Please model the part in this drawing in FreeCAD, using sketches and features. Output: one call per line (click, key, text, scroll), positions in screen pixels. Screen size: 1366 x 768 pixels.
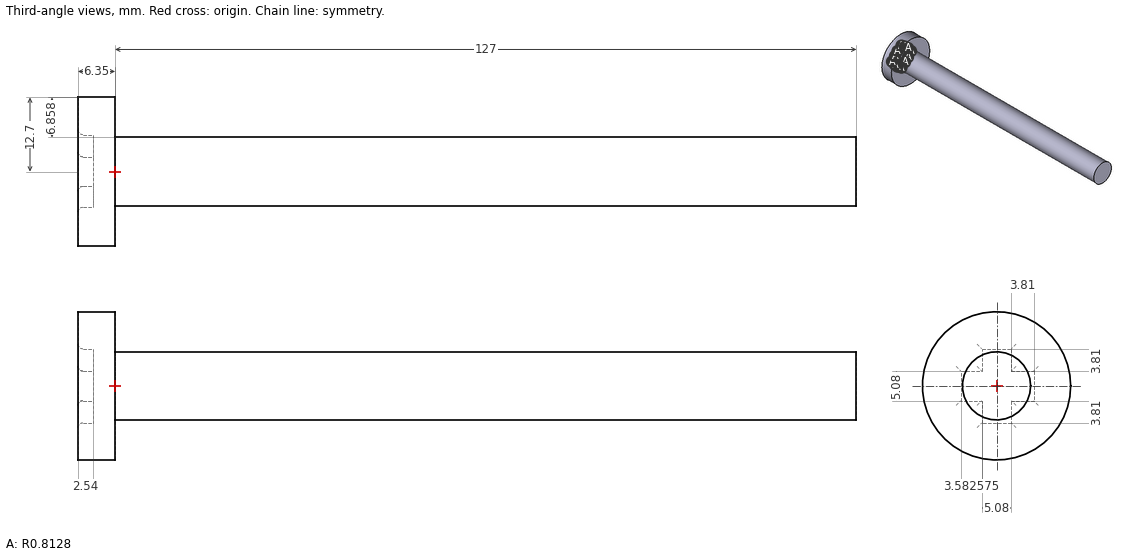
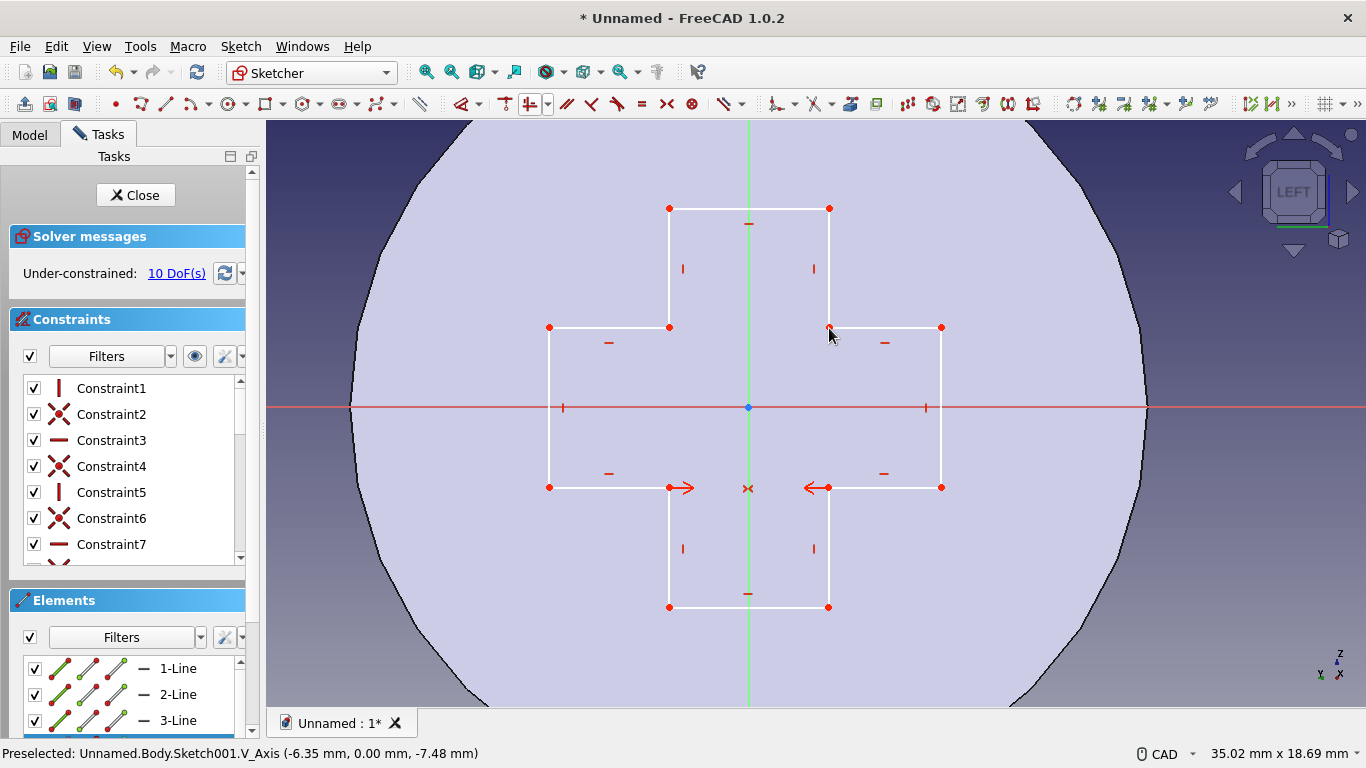
click(359, 407)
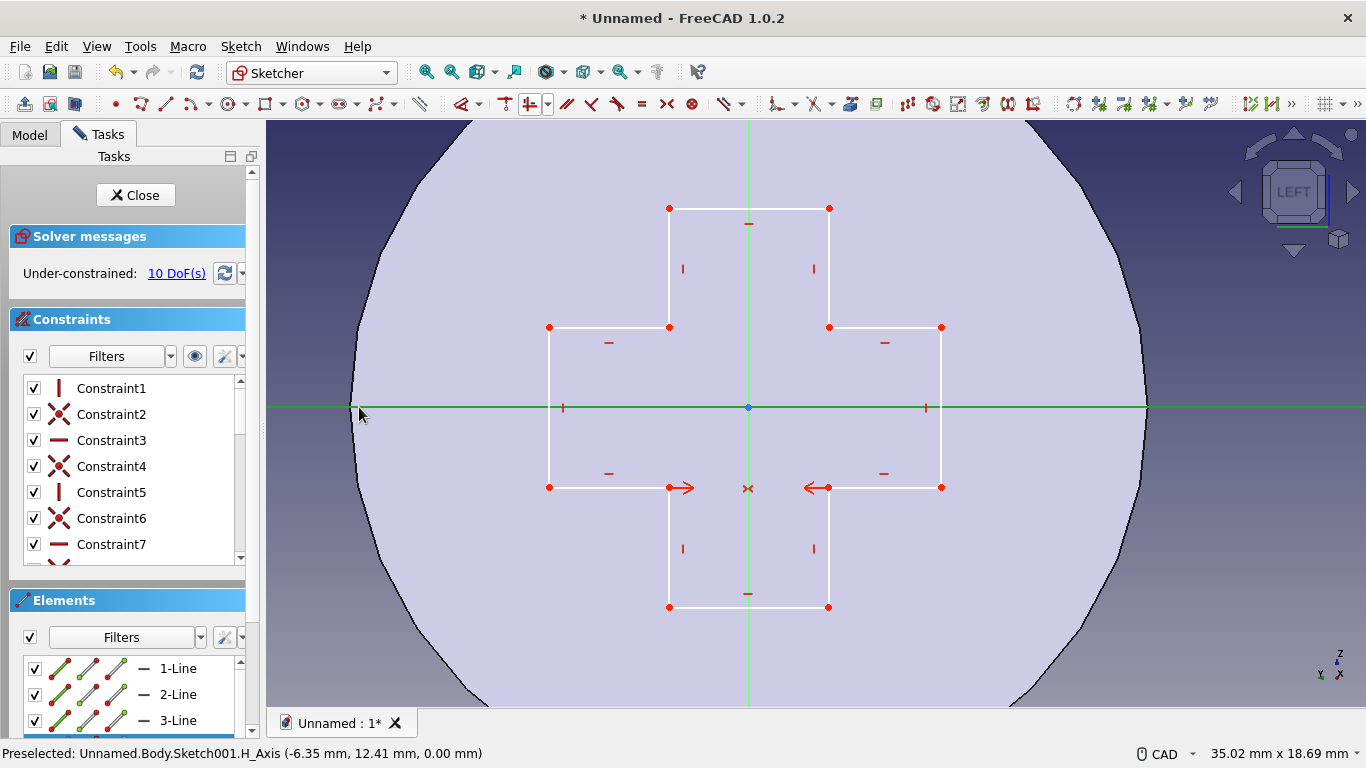
click(667, 104)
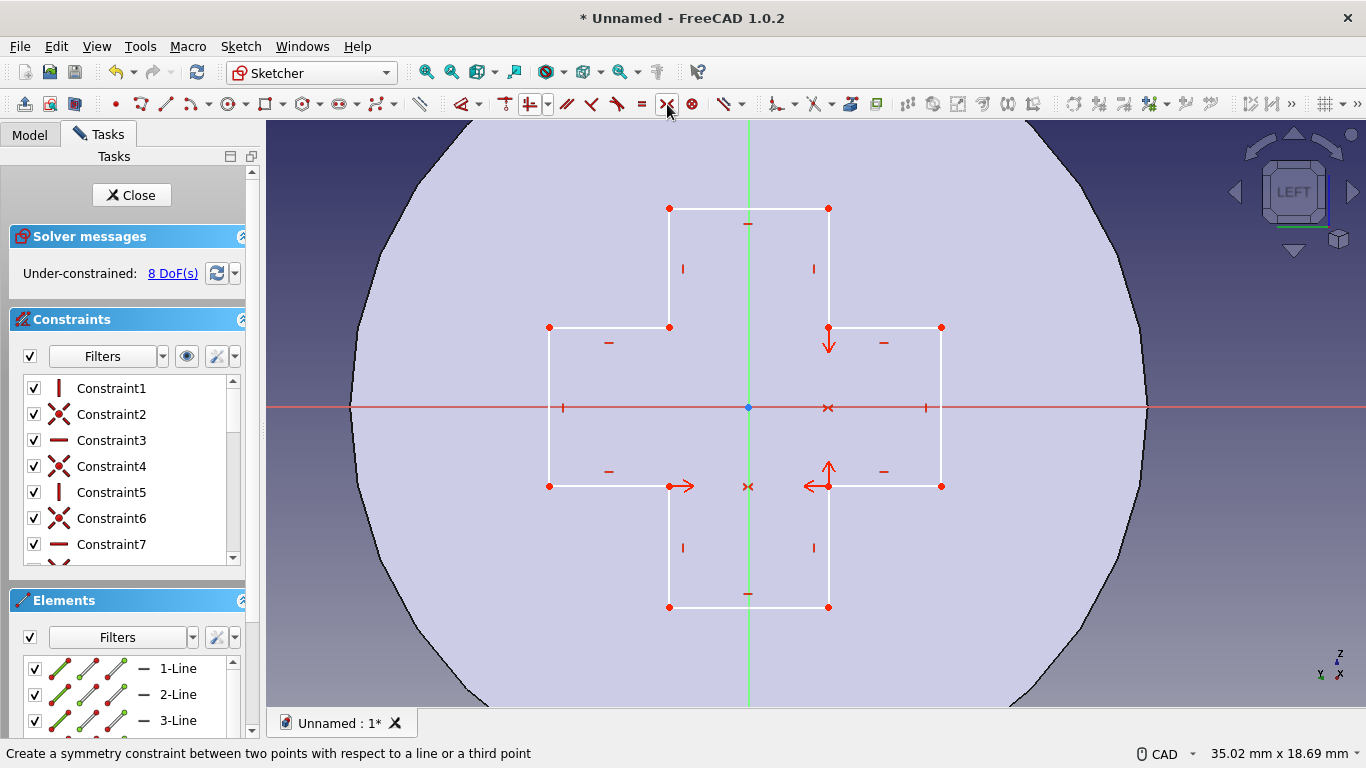
click(669, 608)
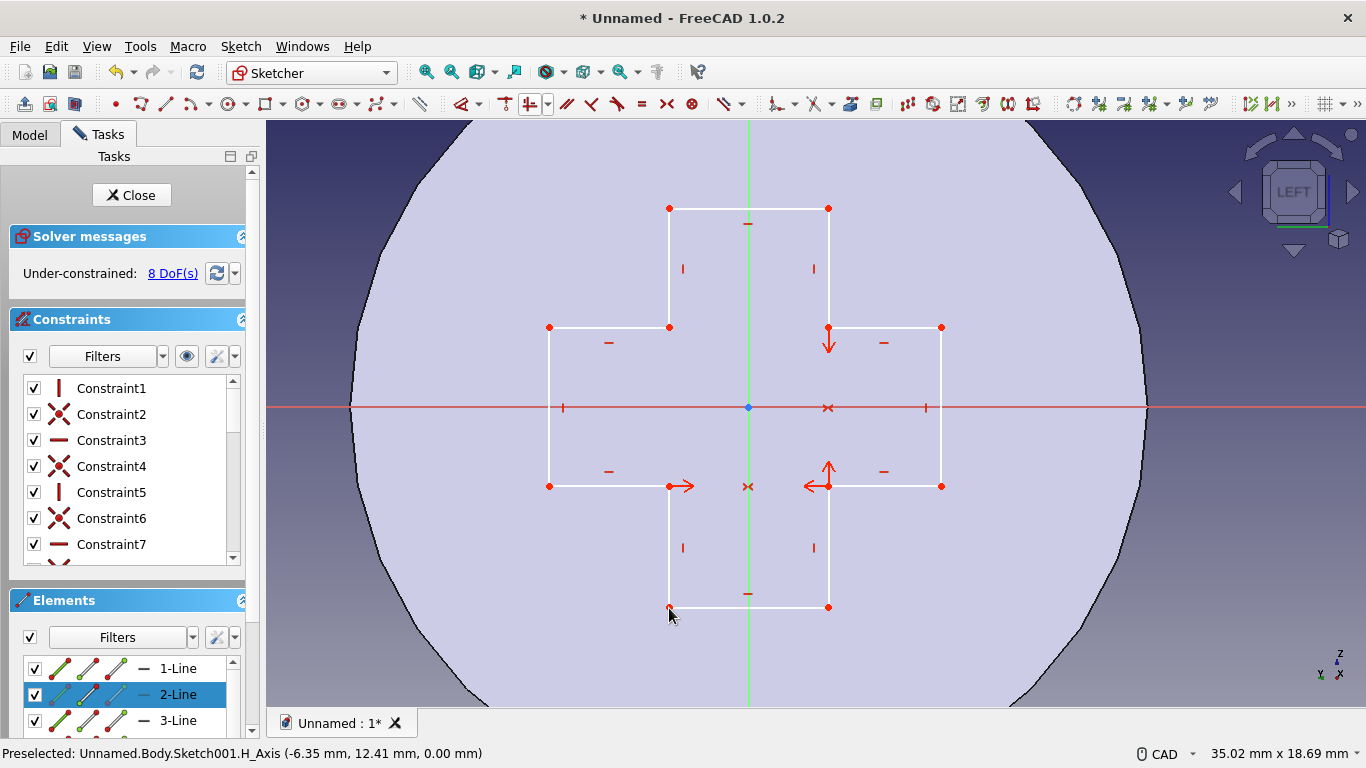
click(669, 209)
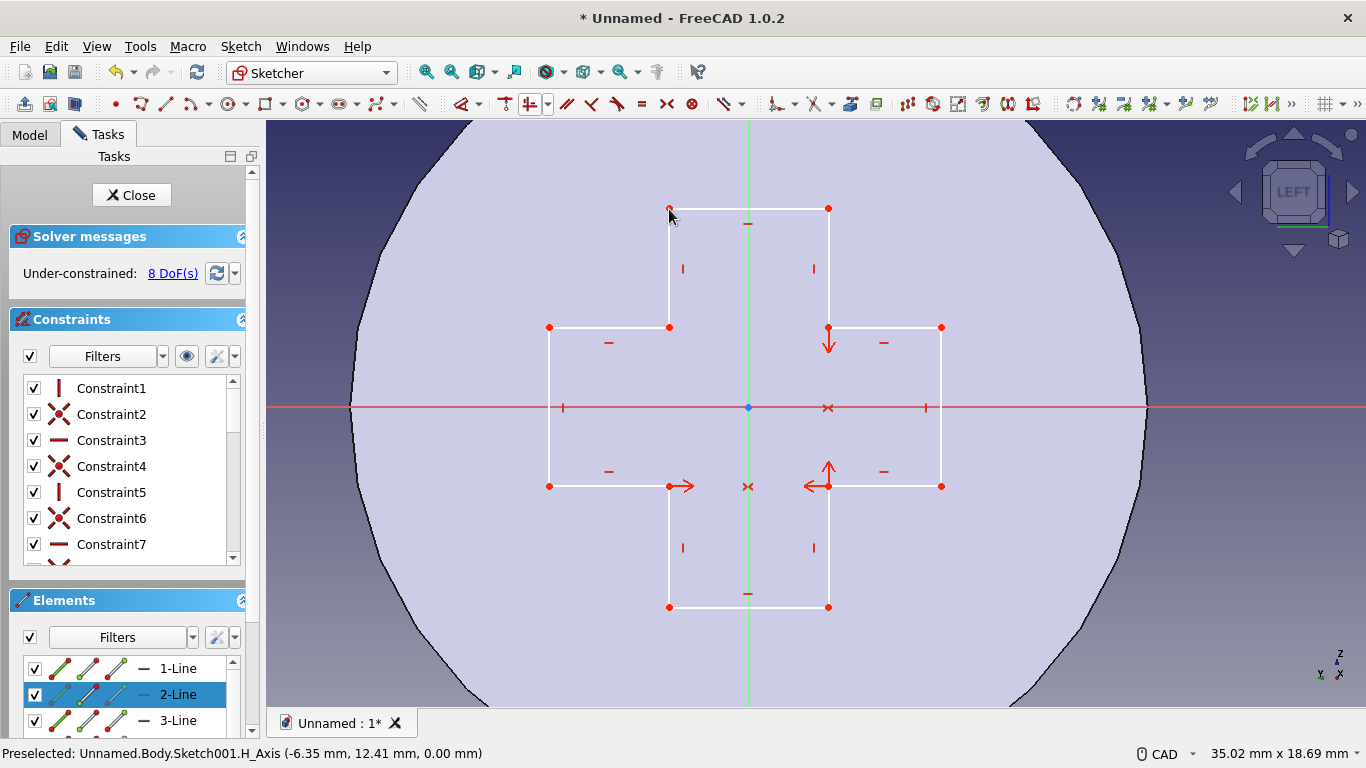
click(359, 407)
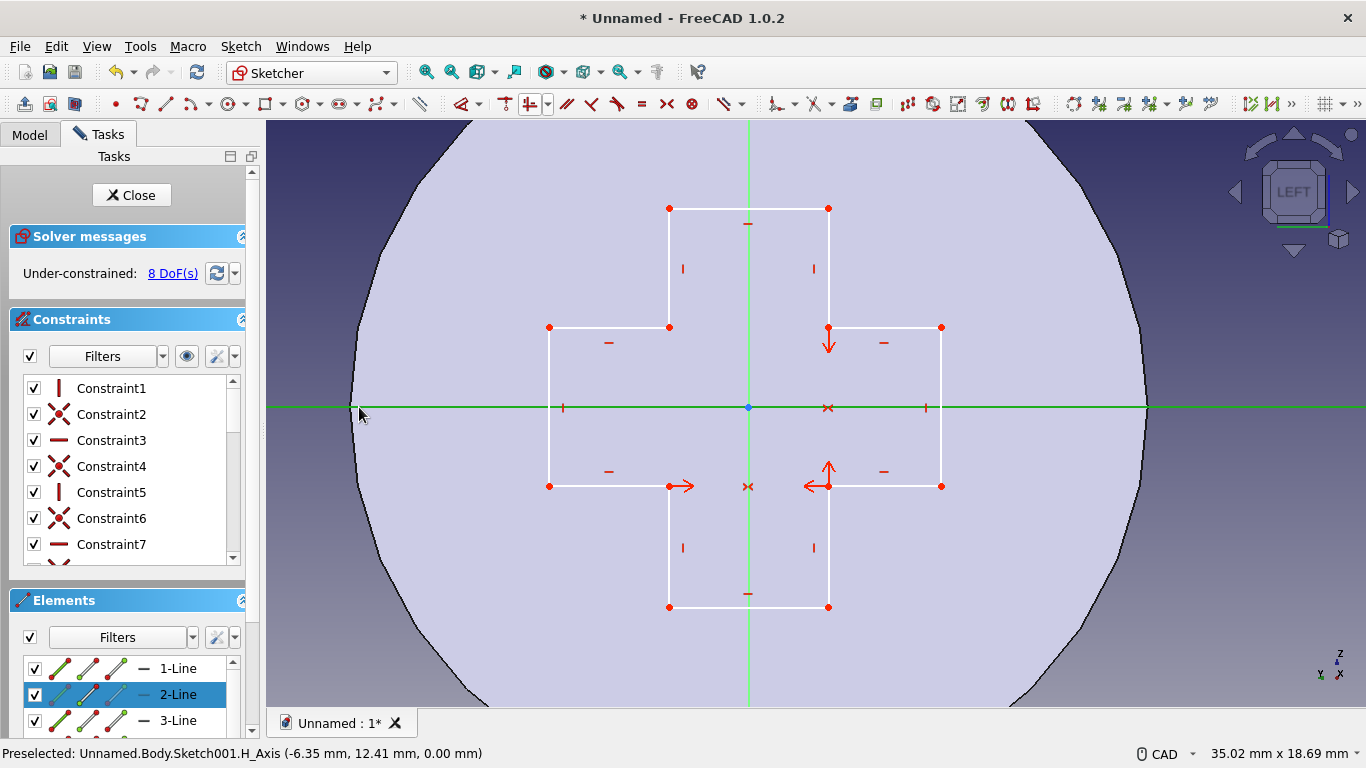
click(667, 104)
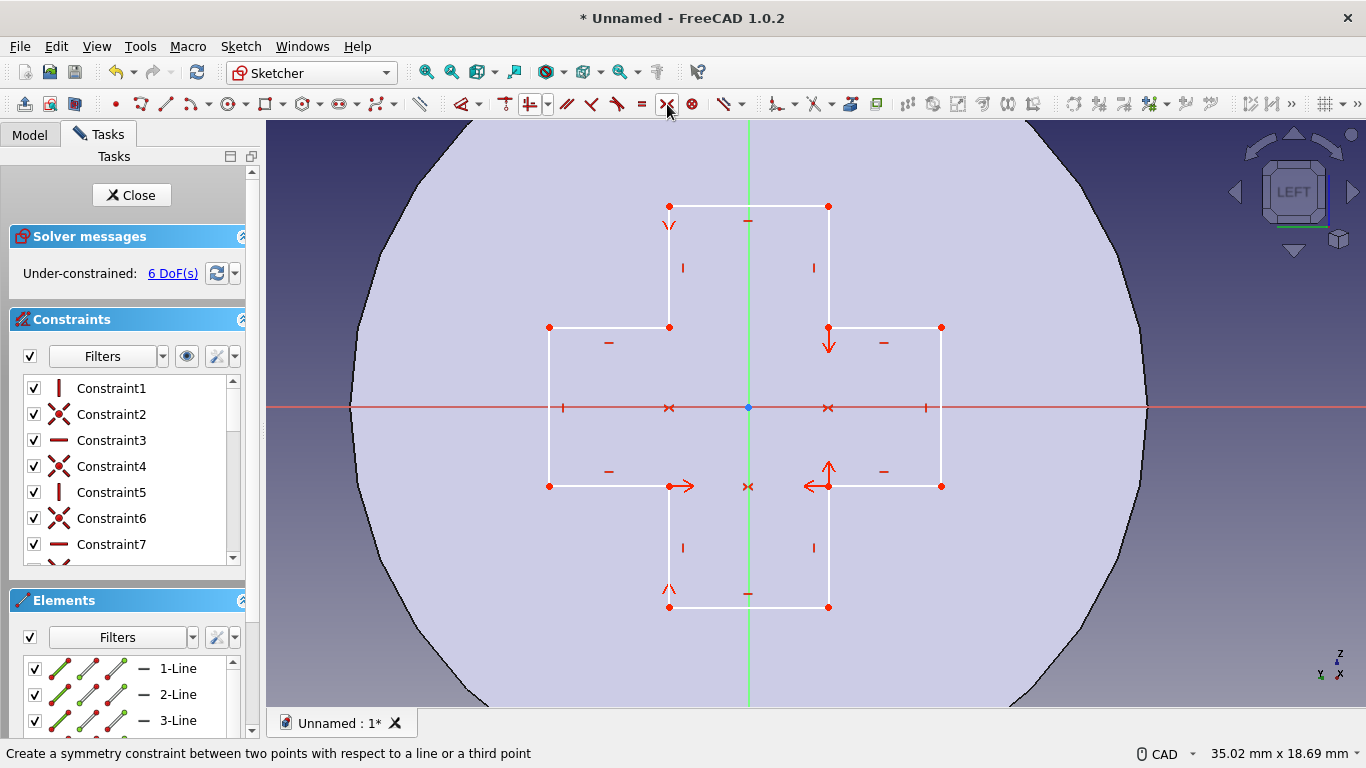
key(d)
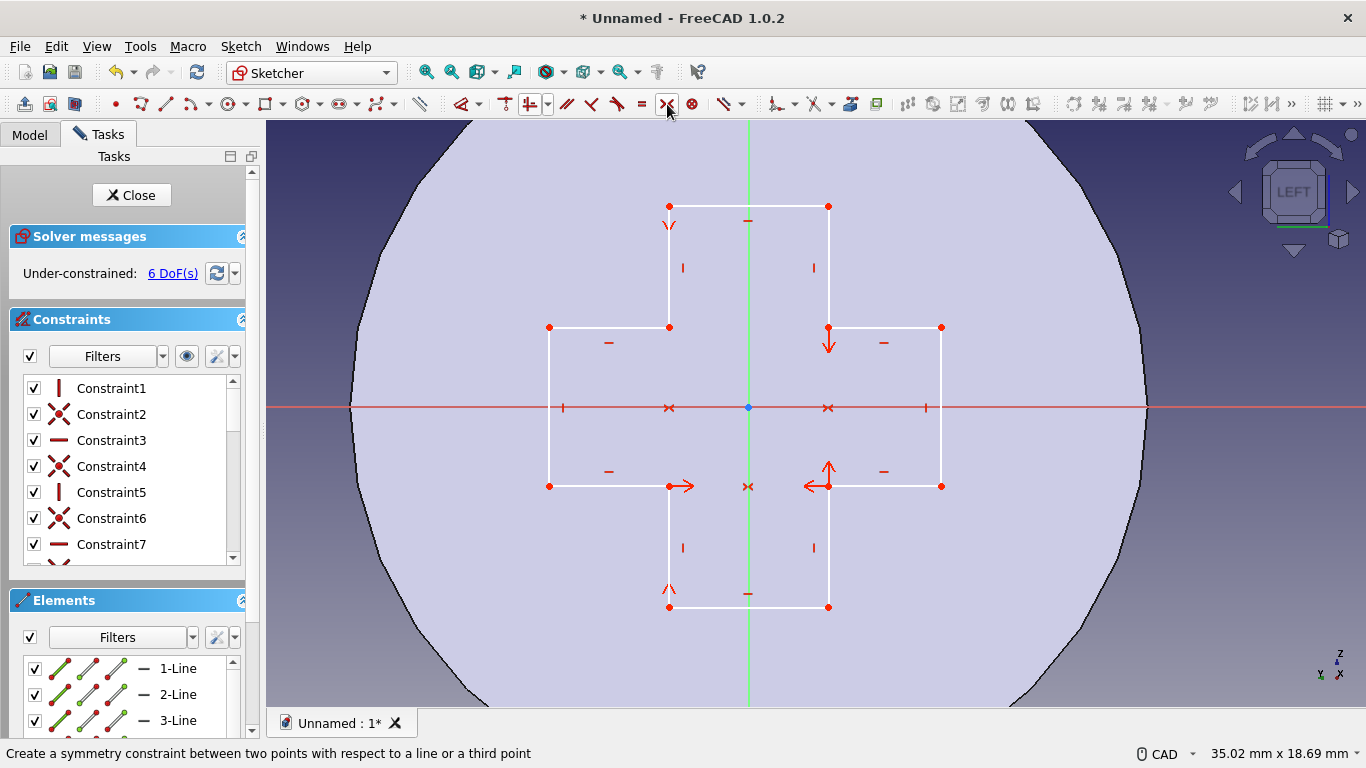
click(669, 523)
click(635, 547)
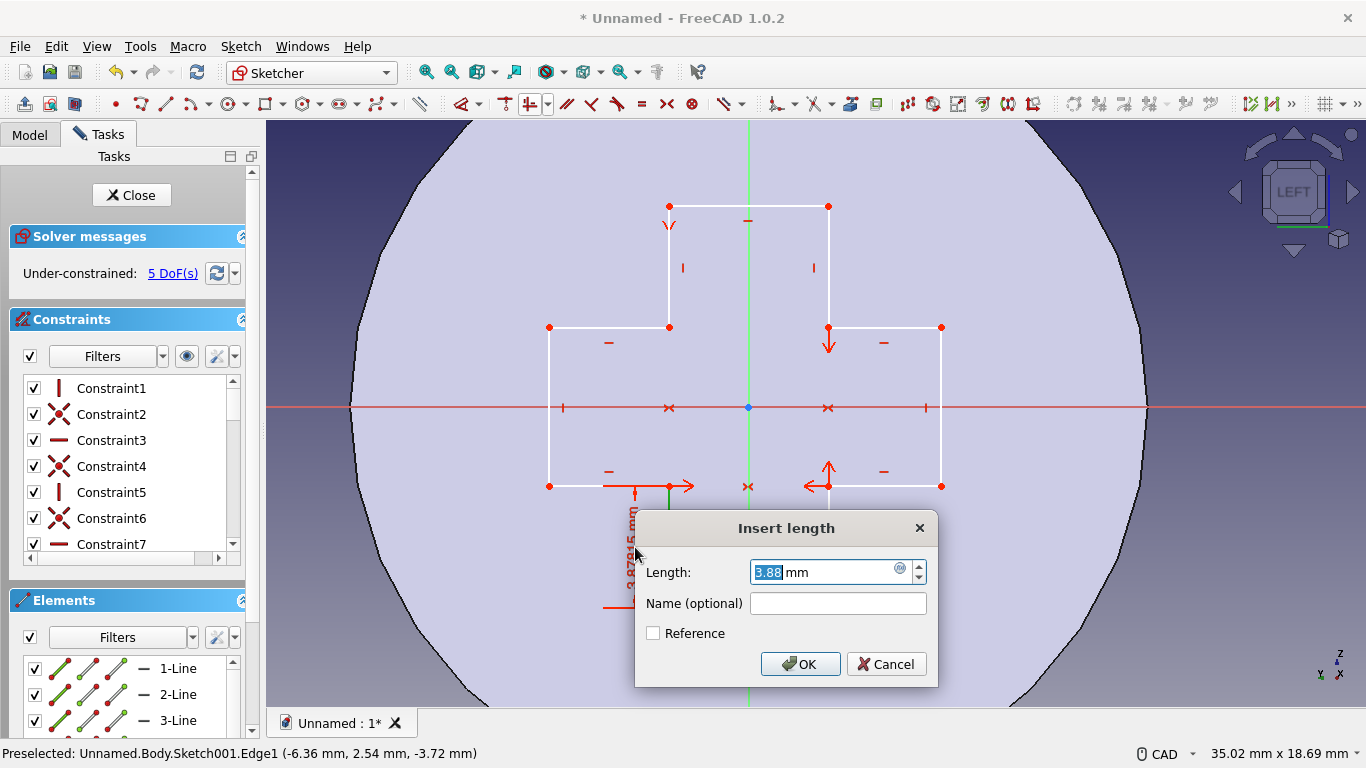
text(3.81)
key(Return)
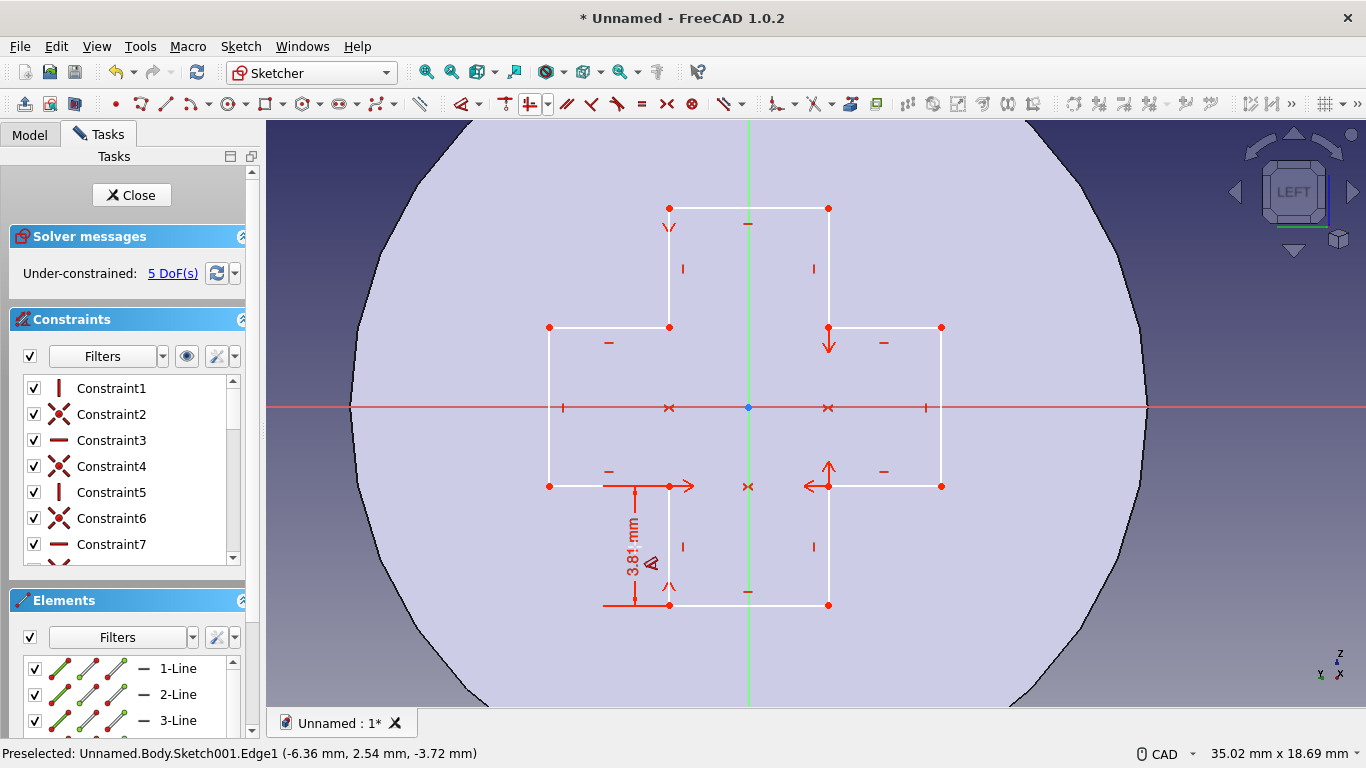
click(717, 606)
click(712, 640)